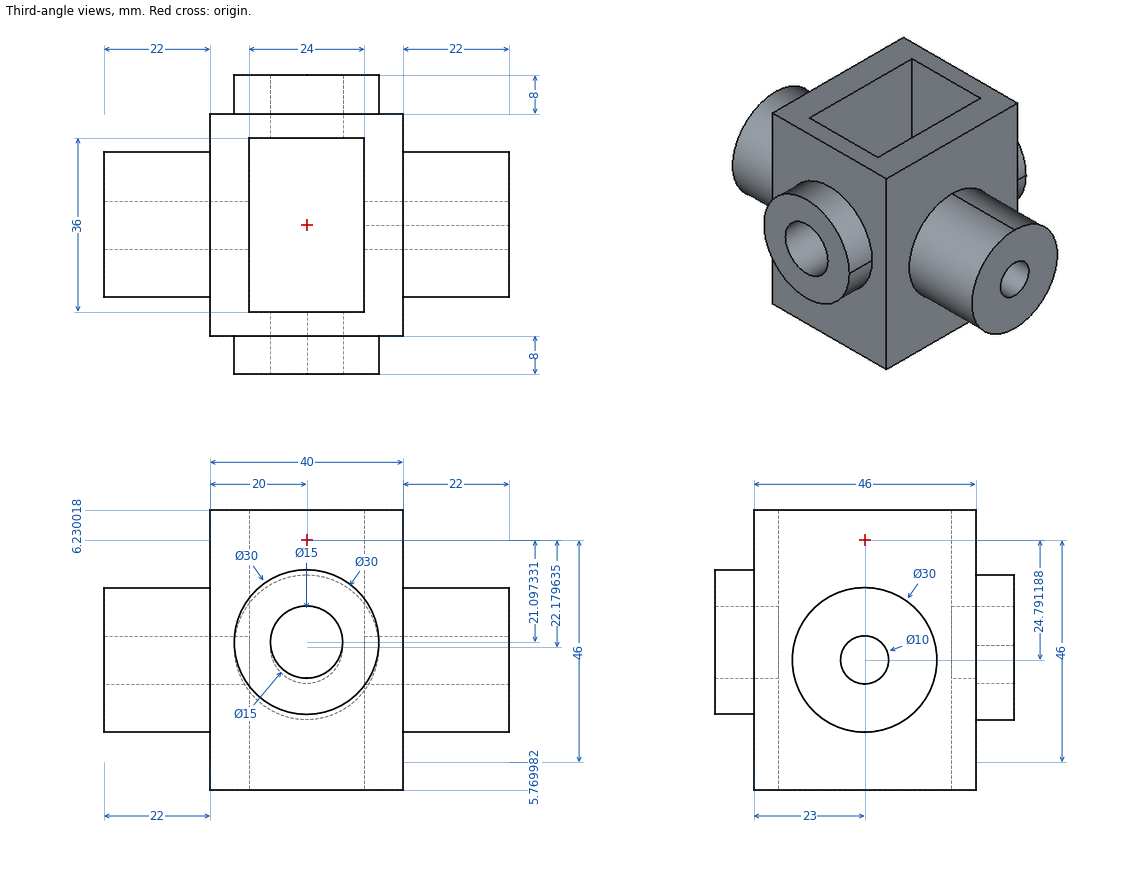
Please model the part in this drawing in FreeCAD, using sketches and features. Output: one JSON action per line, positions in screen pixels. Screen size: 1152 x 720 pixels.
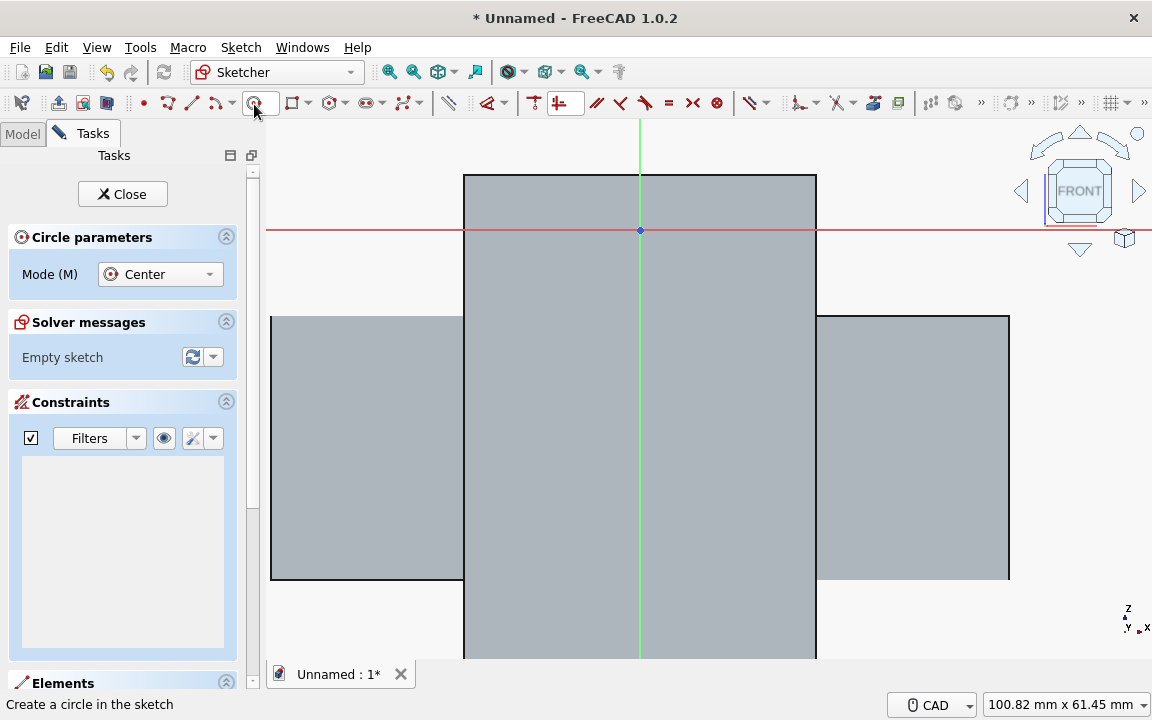
{"action": "left_click", "coordinate": [640, 416]}
{"action": "left_click", "coordinate": [733, 322]}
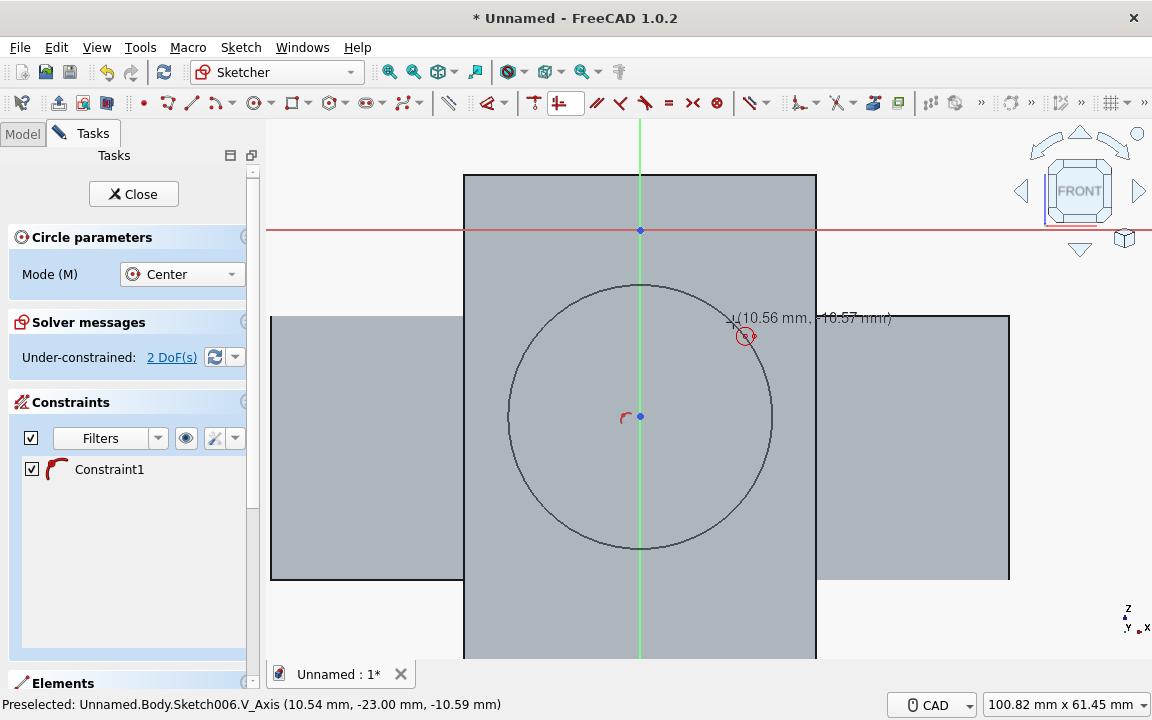
{"action": "left_click", "coordinate": [640, 417]}
{"action": "left_click", "coordinate": [687, 369]}
{"action": "key", "text": "Escape"}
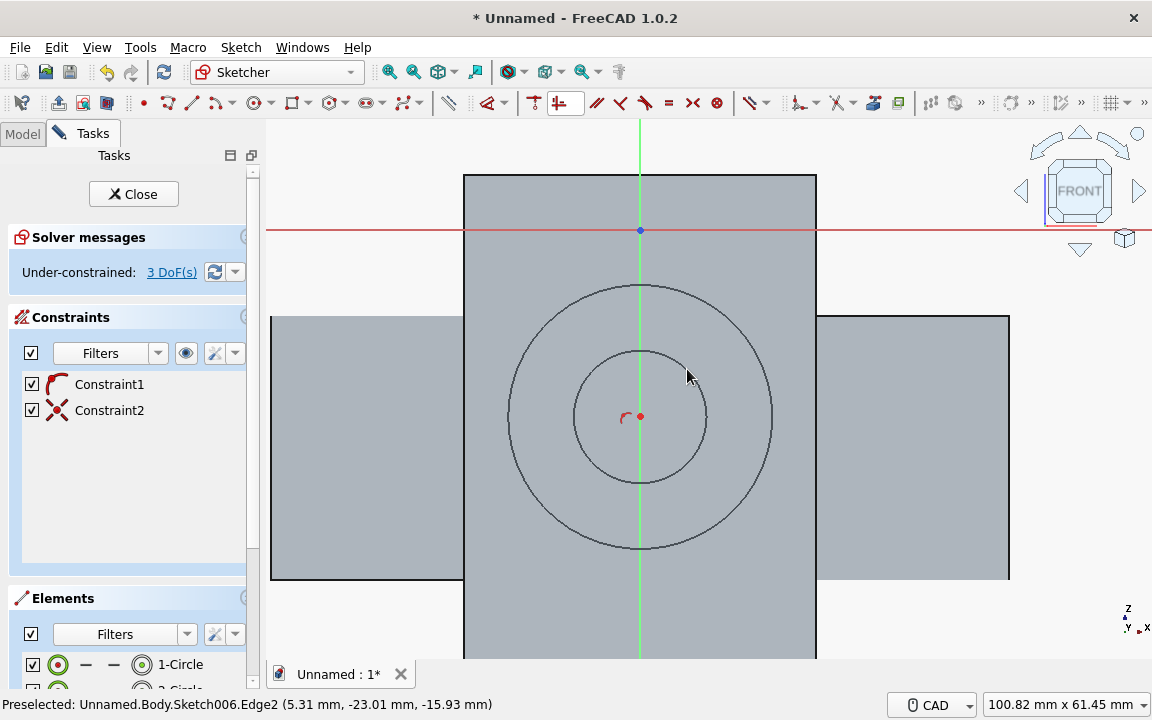
{"action": "left_click", "coordinate": [488, 104]}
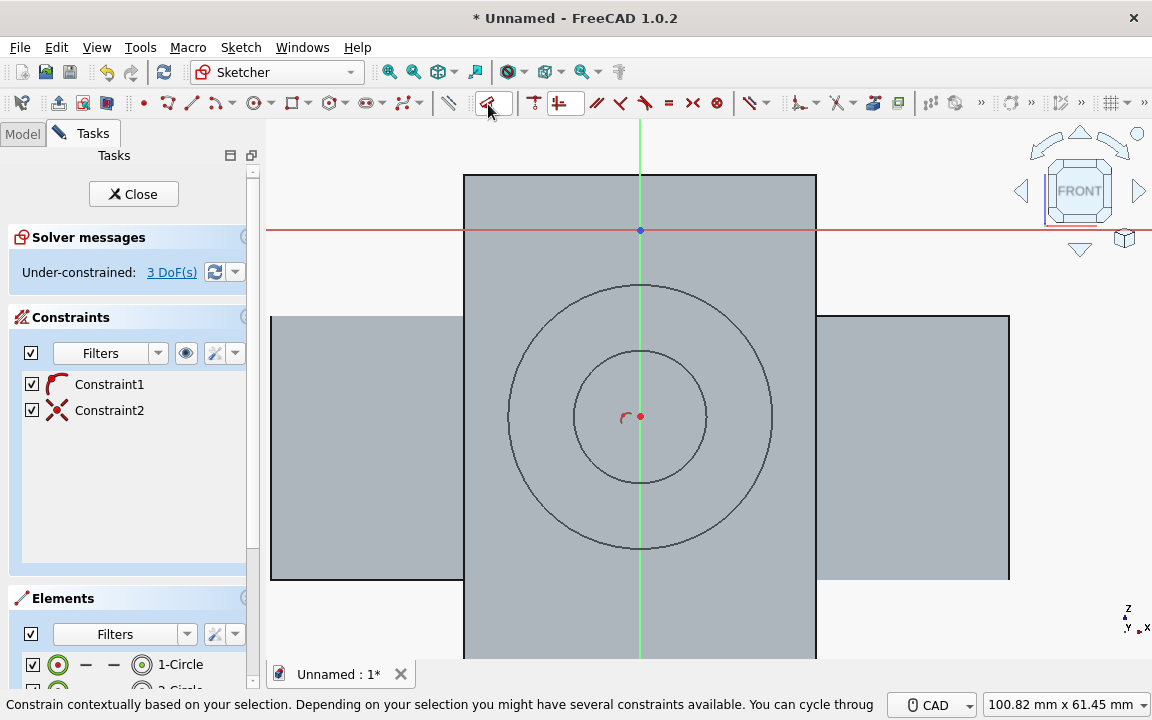
{"action": "left_click", "coordinate": [733, 323]}
{"action": "left_click", "coordinate": [755, 300]}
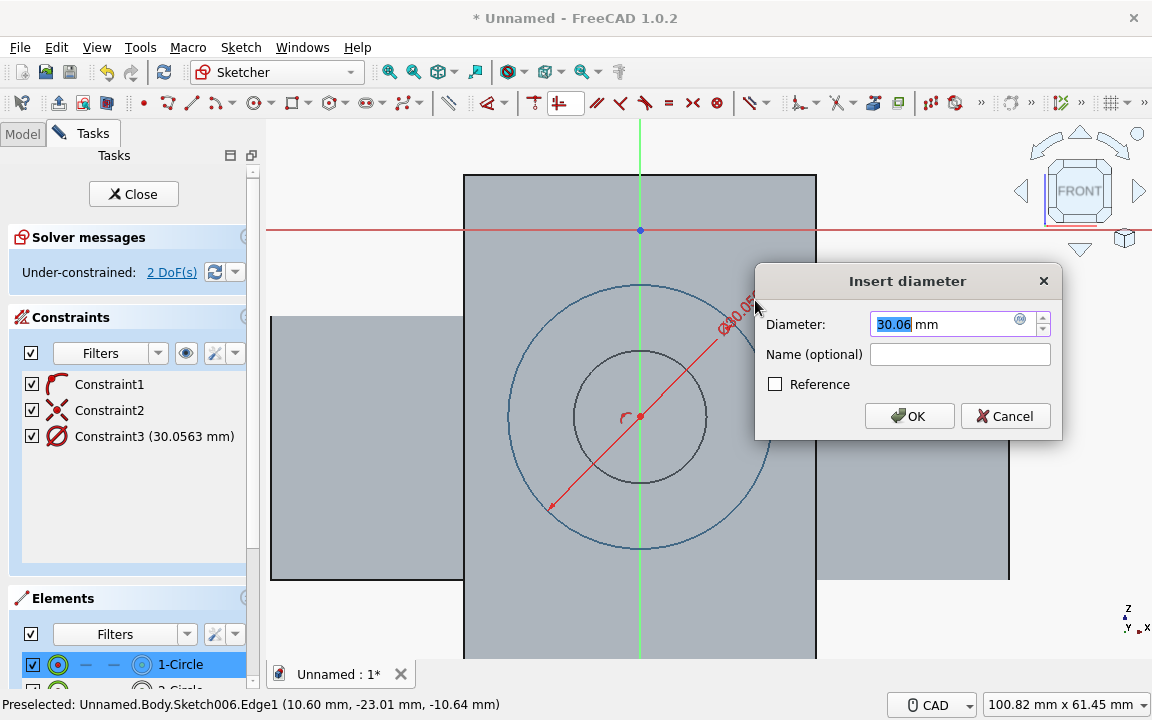
{"action": "type", "text": "30"}
{"action": "key", "text": "Return"}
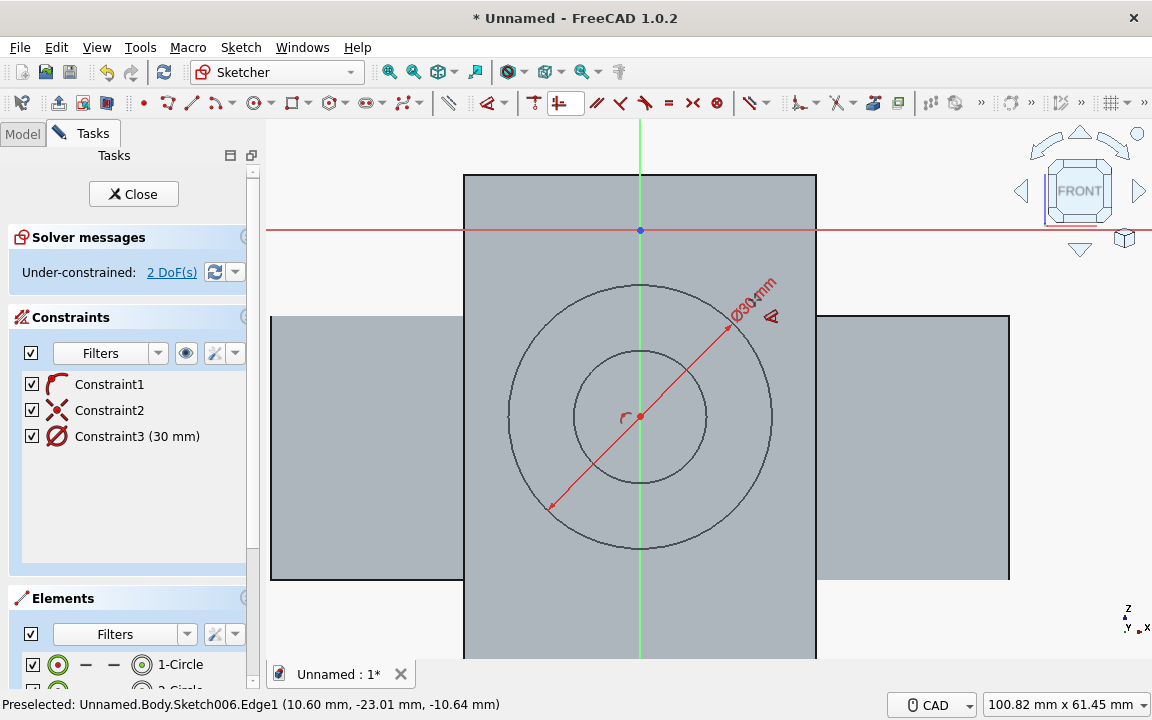
{"action": "left_click", "coordinate": [687, 370]}
{"action": "left_click", "coordinate": [710, 347]}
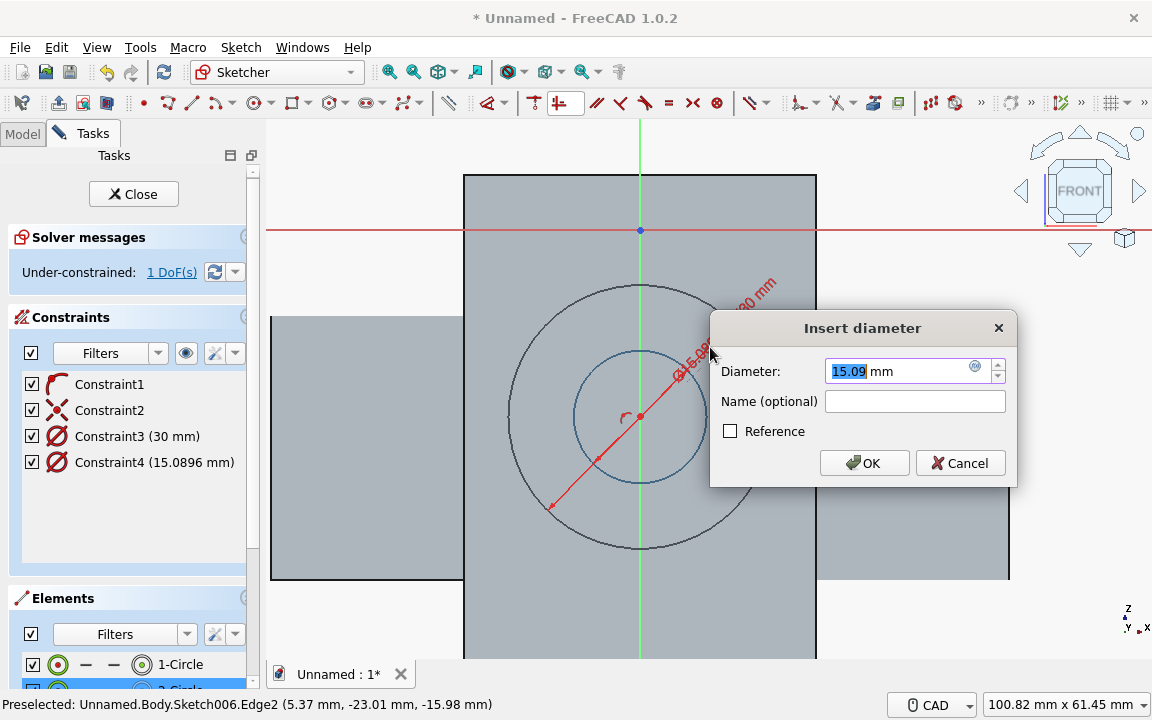
{"action": "type", "text": "15"}
{"action": "key", "text": "Return"}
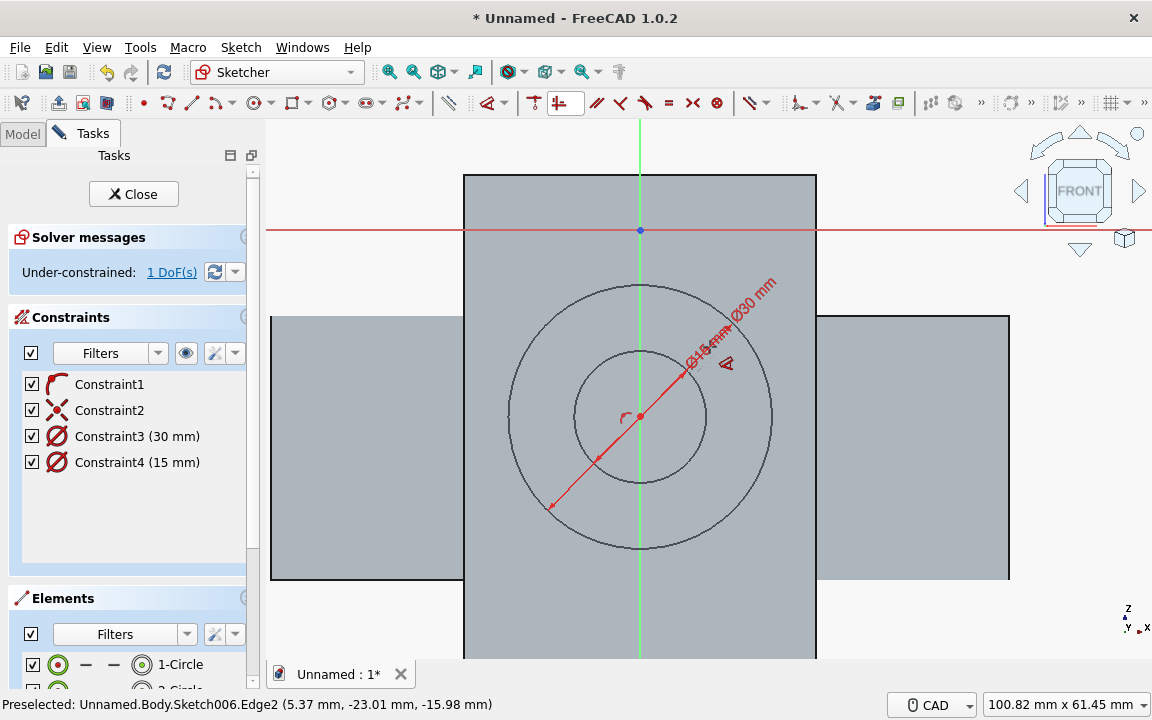
{"action": "left_click", "coordinate": [640, 417]}
{"action": "left_click", "coordinate": [674, 324]}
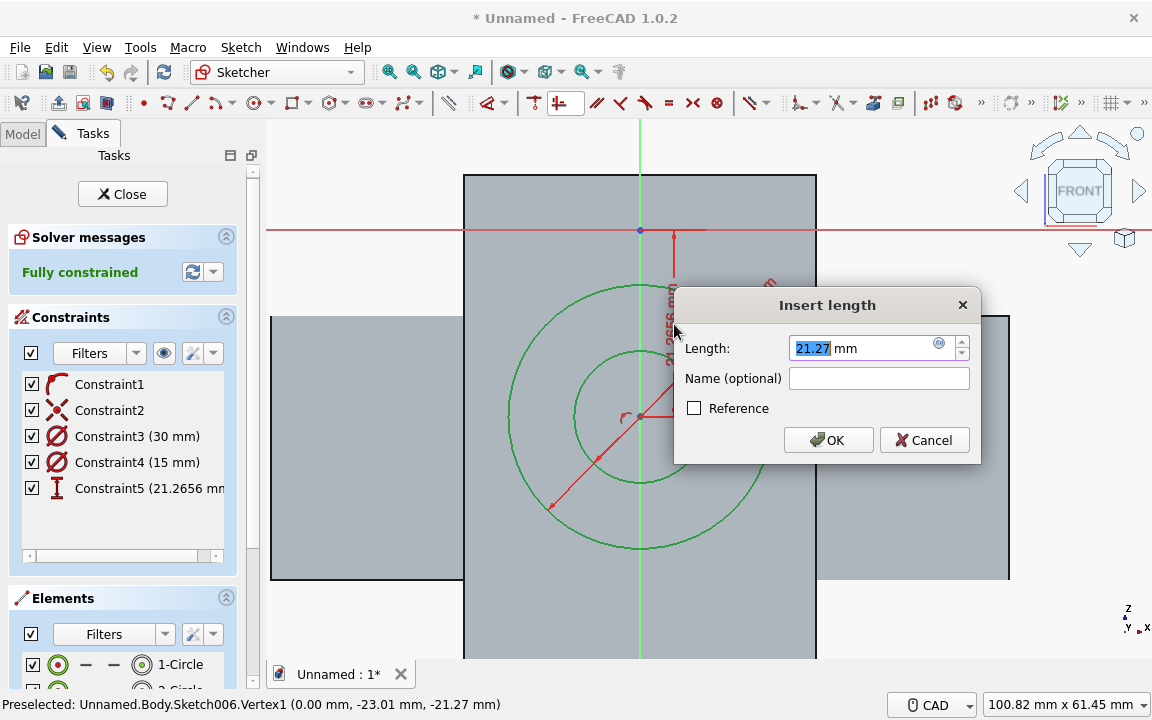
{"action": "type", "text": "21.097331"}
{"action": "key", "text": "Return"}
{"action": "key", "text": "Escape"}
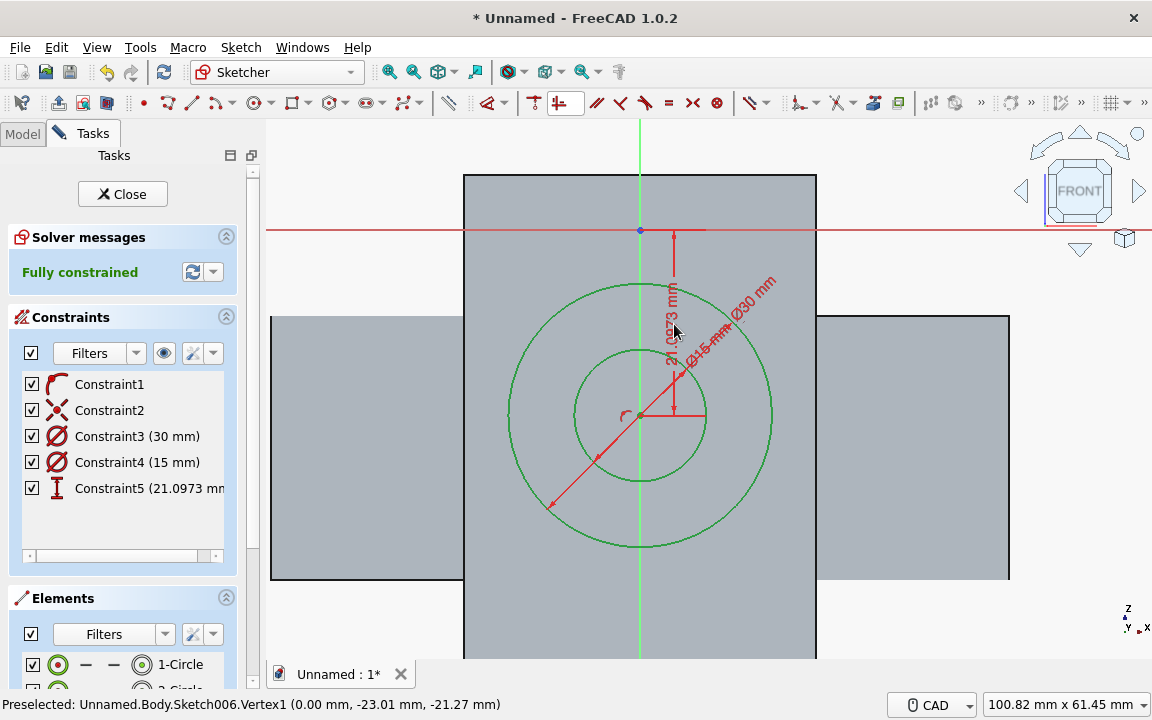
{"action": "left_click", "coordinate": [123, 194]}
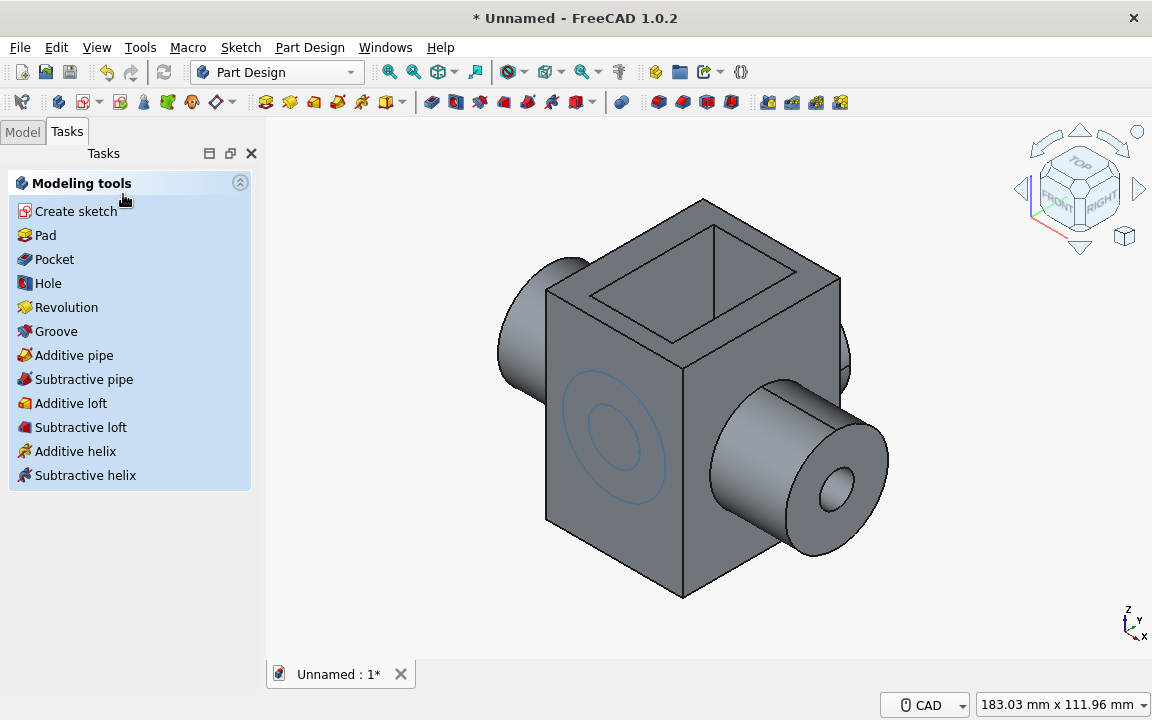
{"action": "left_click", "coordinate": [266, 102]}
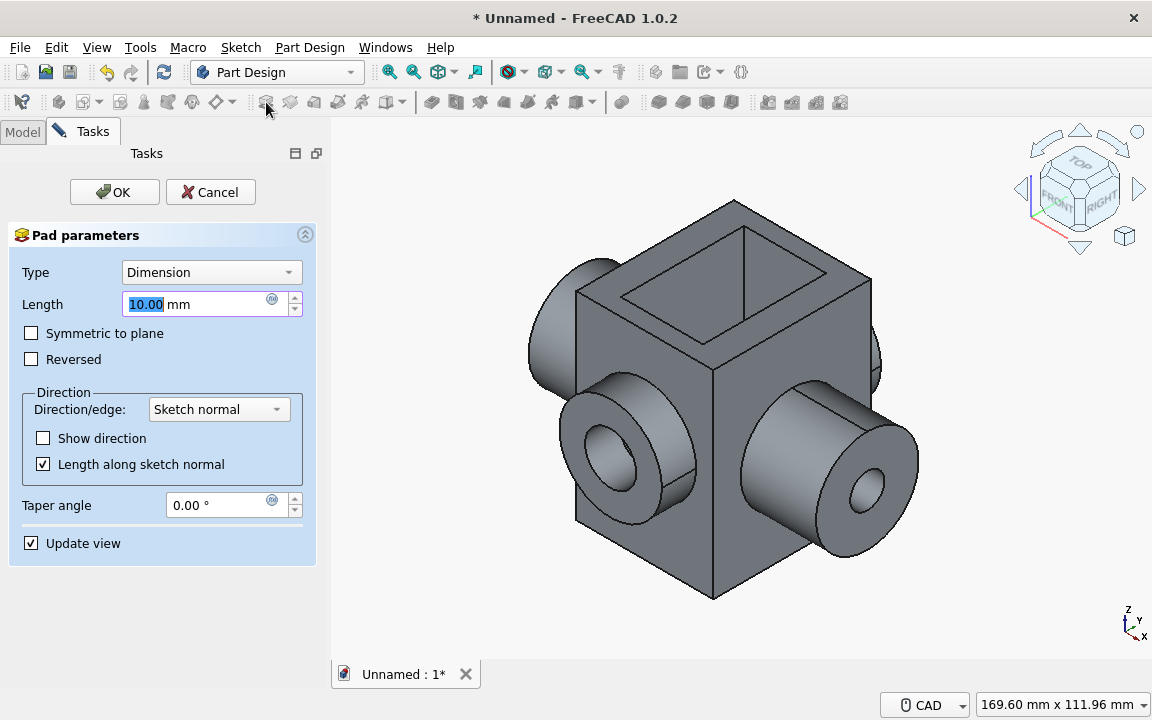
{"action": "type", "text": "8"}
{"action": "key", "text": "Tab"}